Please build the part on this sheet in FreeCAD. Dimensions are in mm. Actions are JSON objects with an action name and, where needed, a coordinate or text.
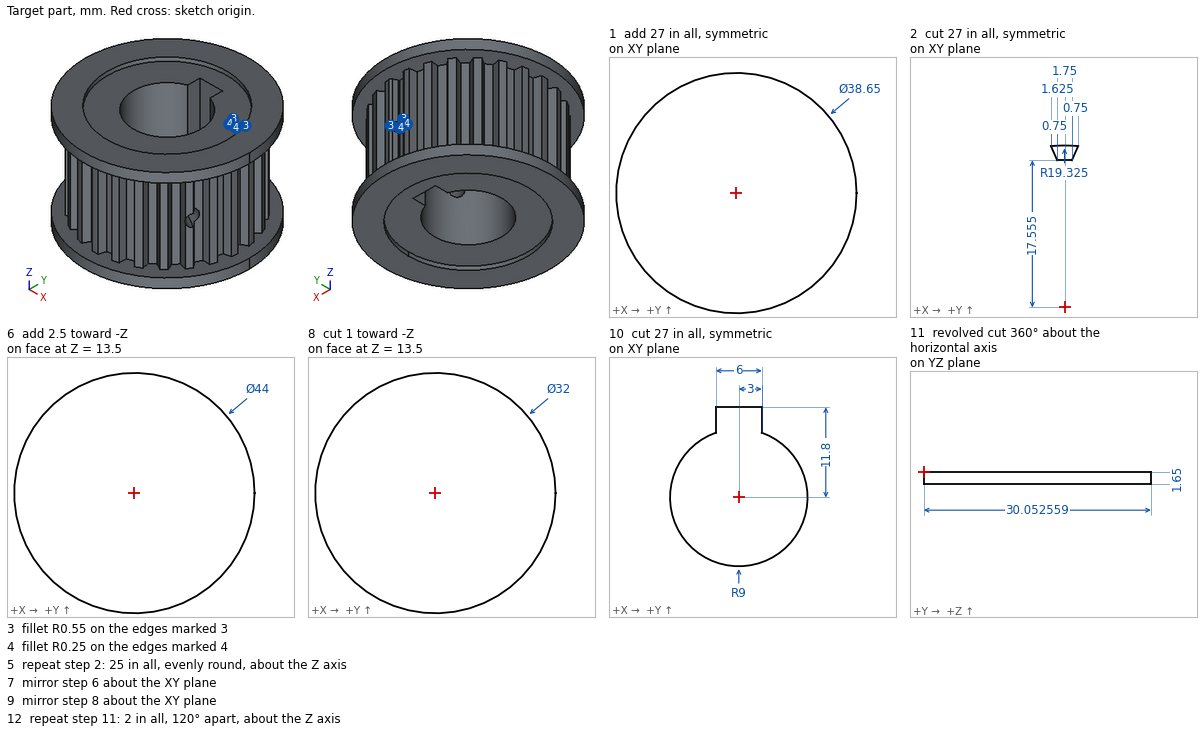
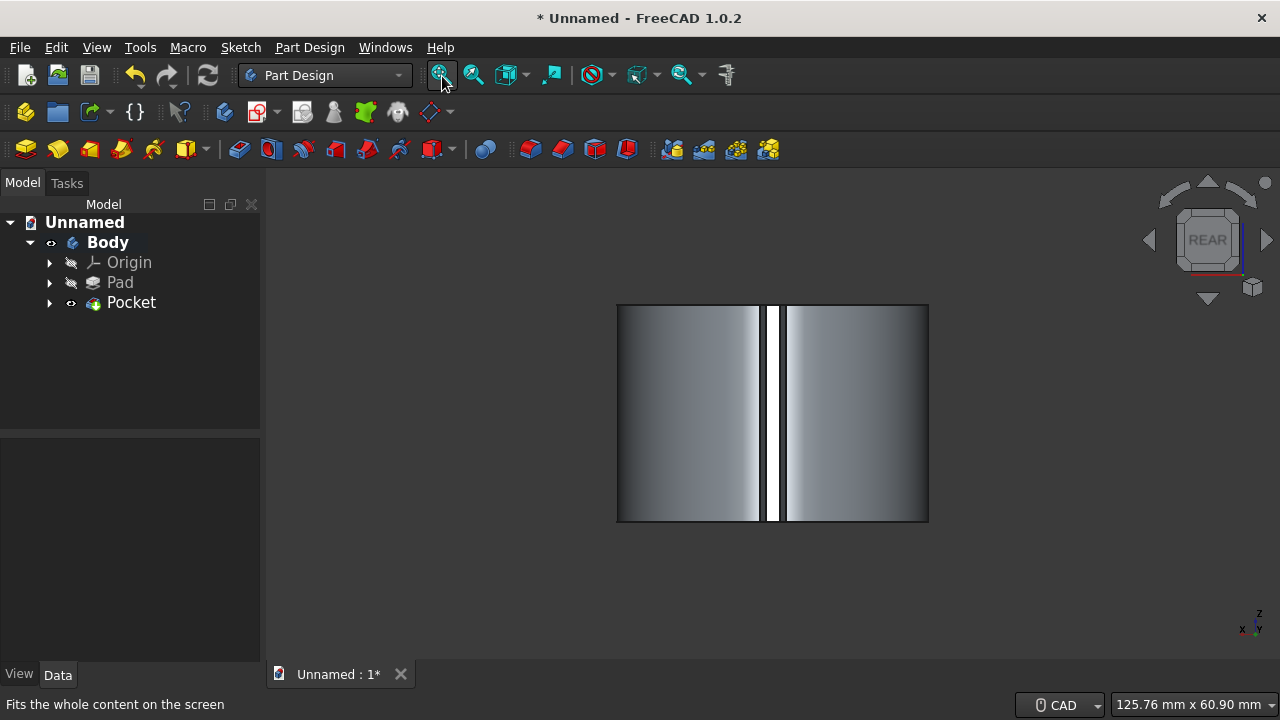
{"action": "left_click", "coordinate": [442, 76]}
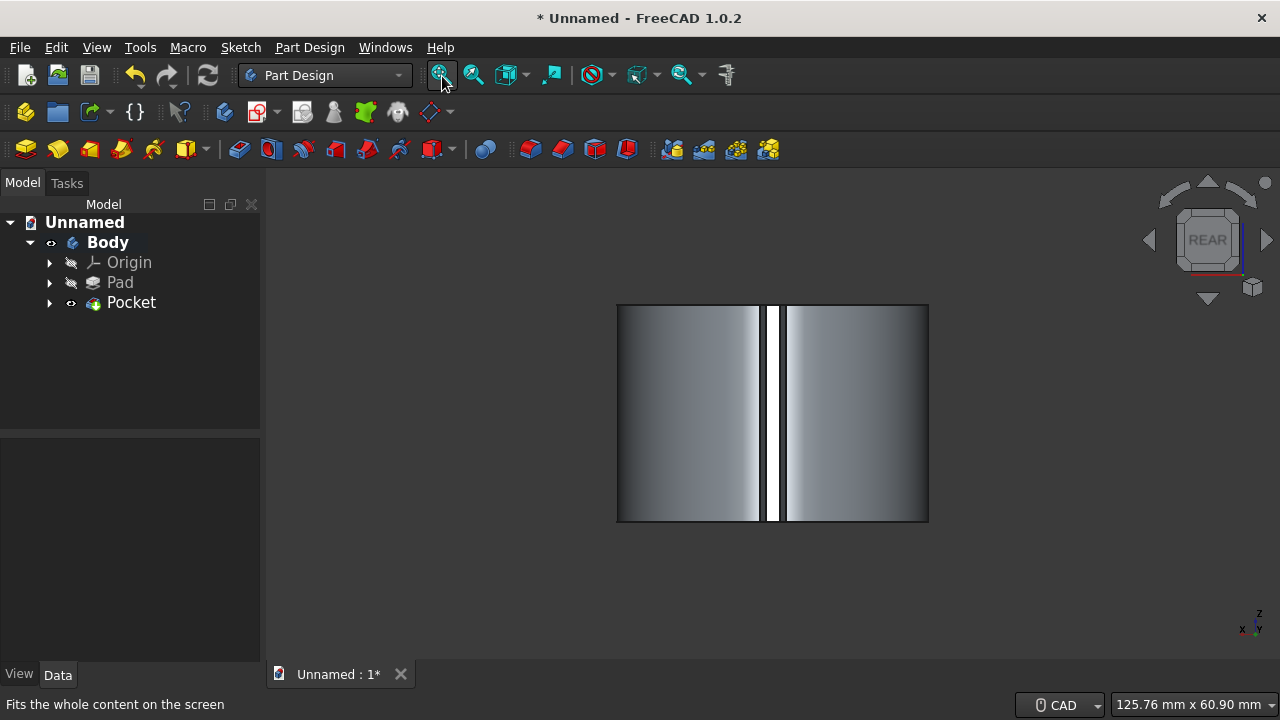
{"action": "left_click", "coordinate": [786, 413]}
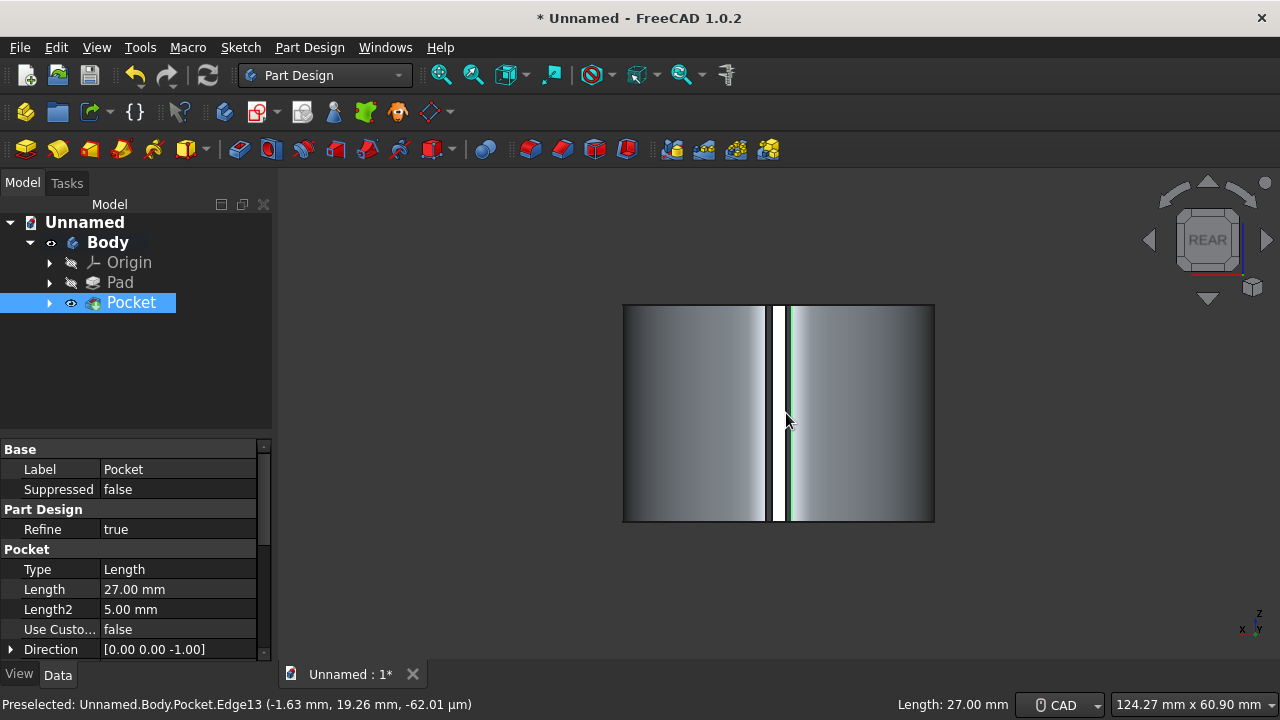
{"action": "left_click", "coordinate": [766, 413], "text": "ctrl"}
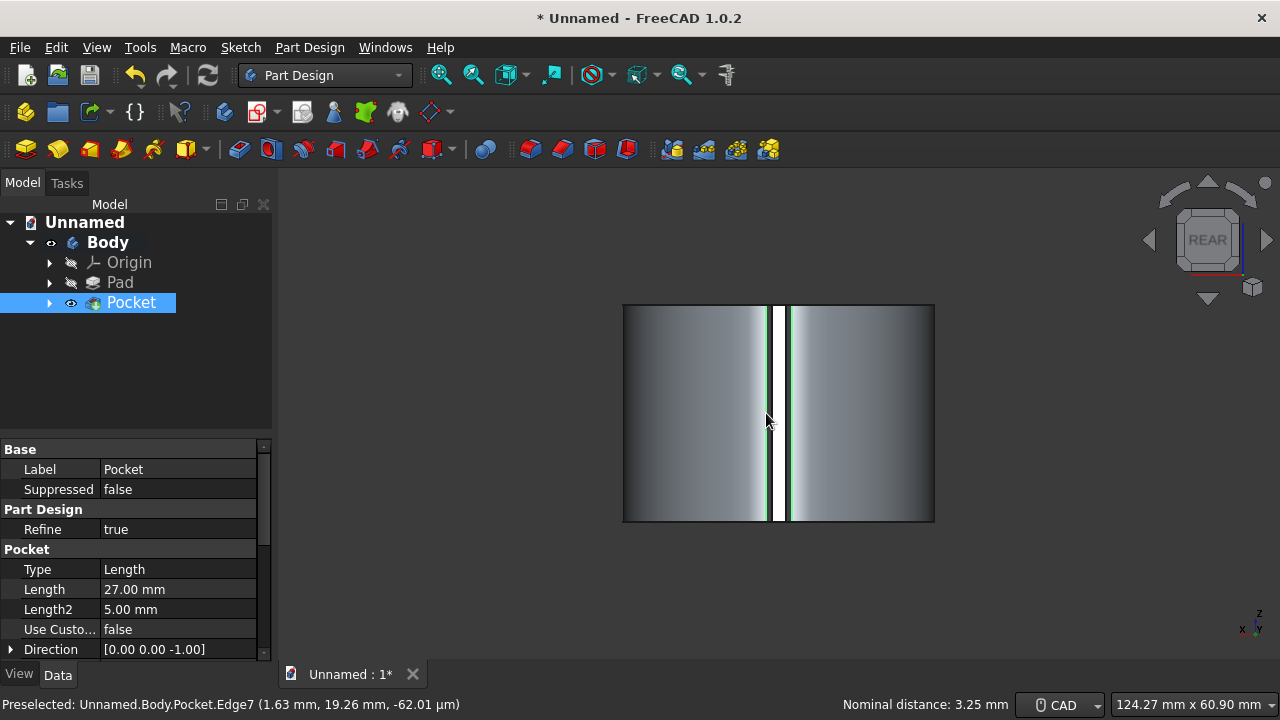
{"action": "left_click", "coordinate": [532, 150]}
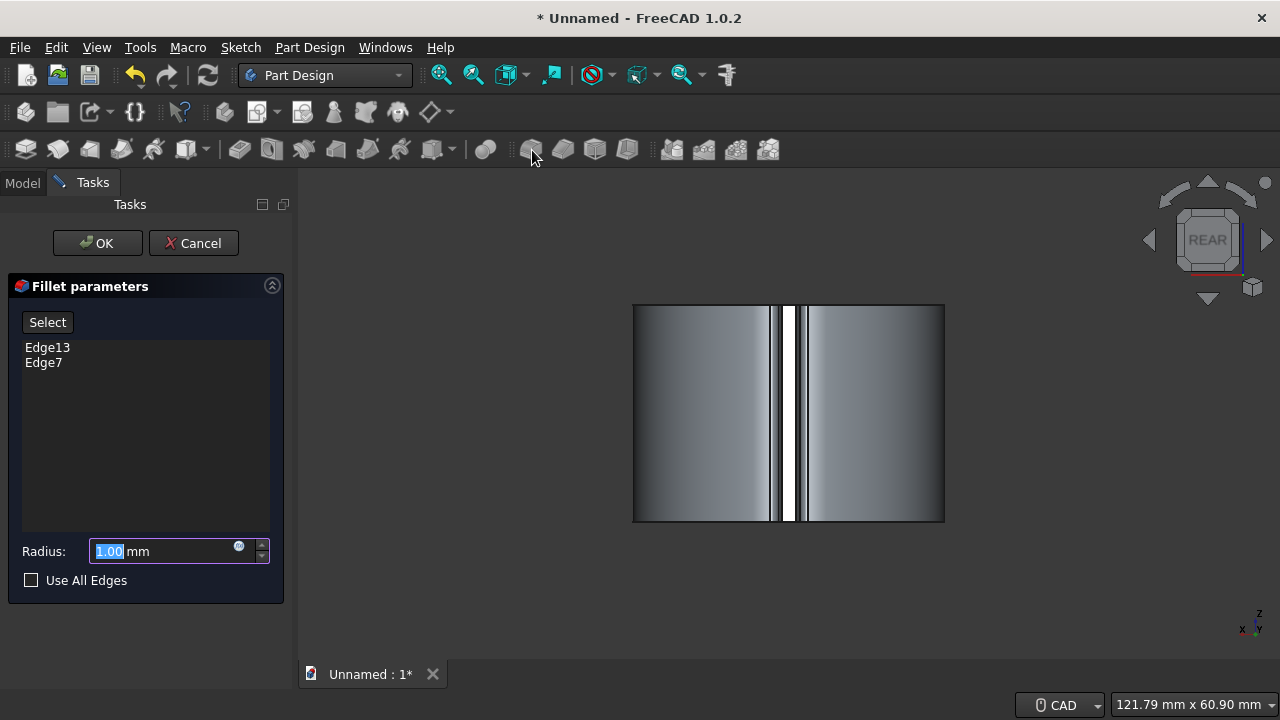
{"action": "type", "text": "0.55"}
{"action": "key", "text": "Tab"}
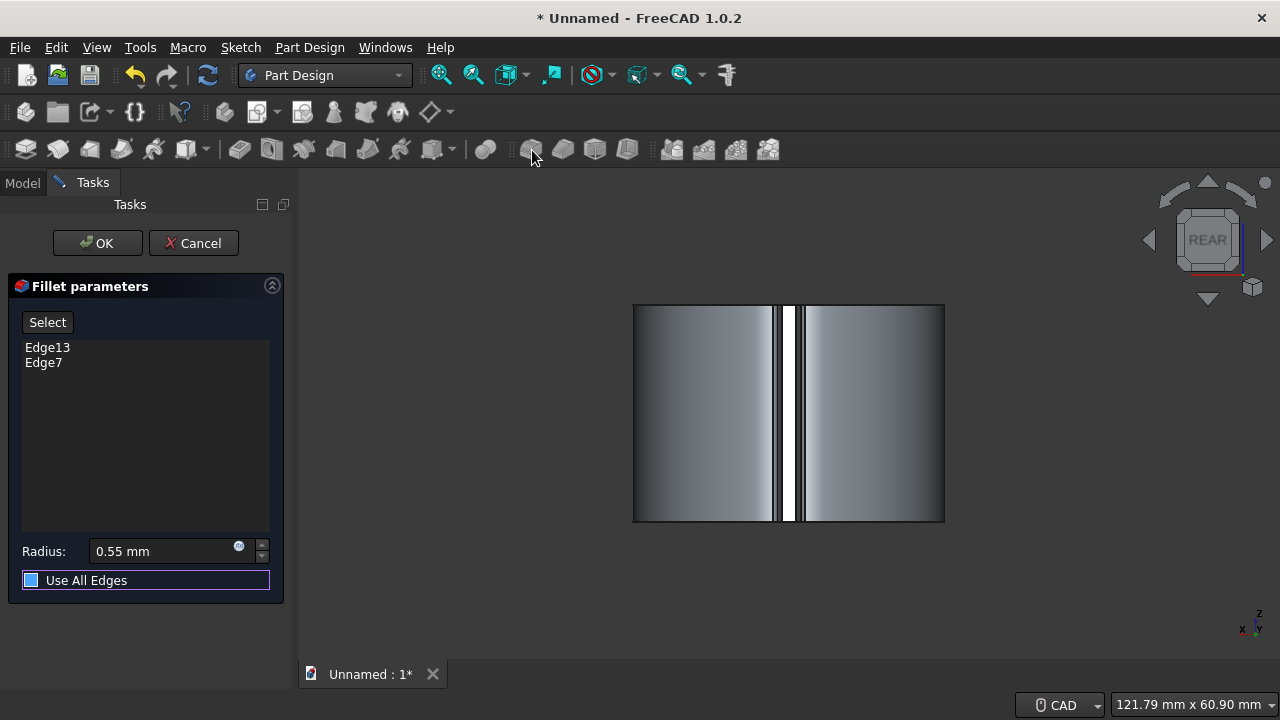
{"action": "left_click", "coordinate": [98, 243]}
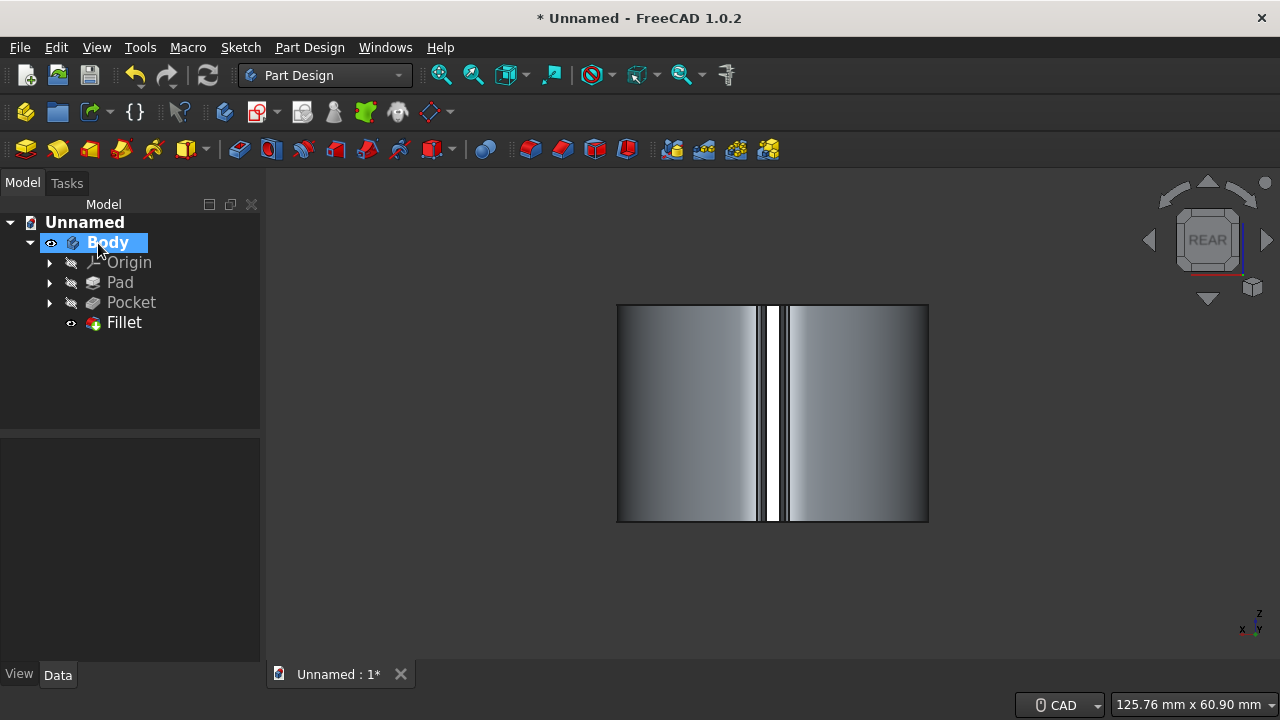
{"action": "left_click", "coordinate": [442, 76]}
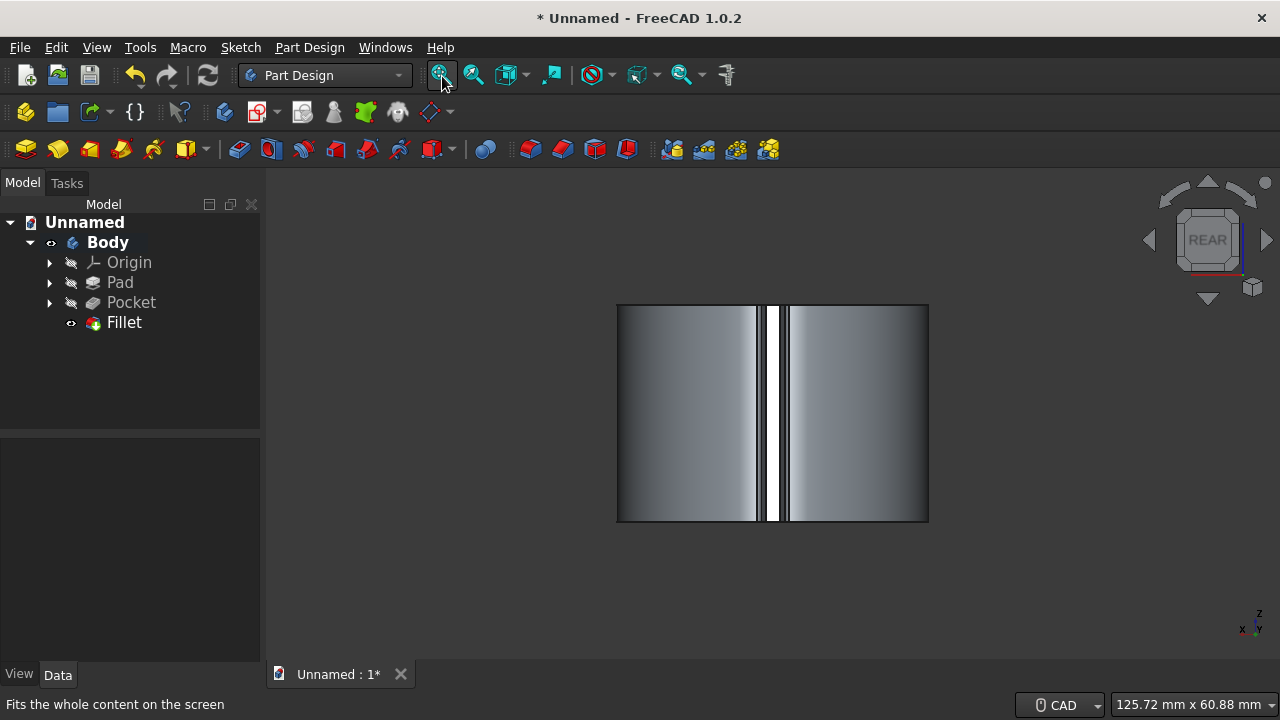
{"action": "key", "text": "0"}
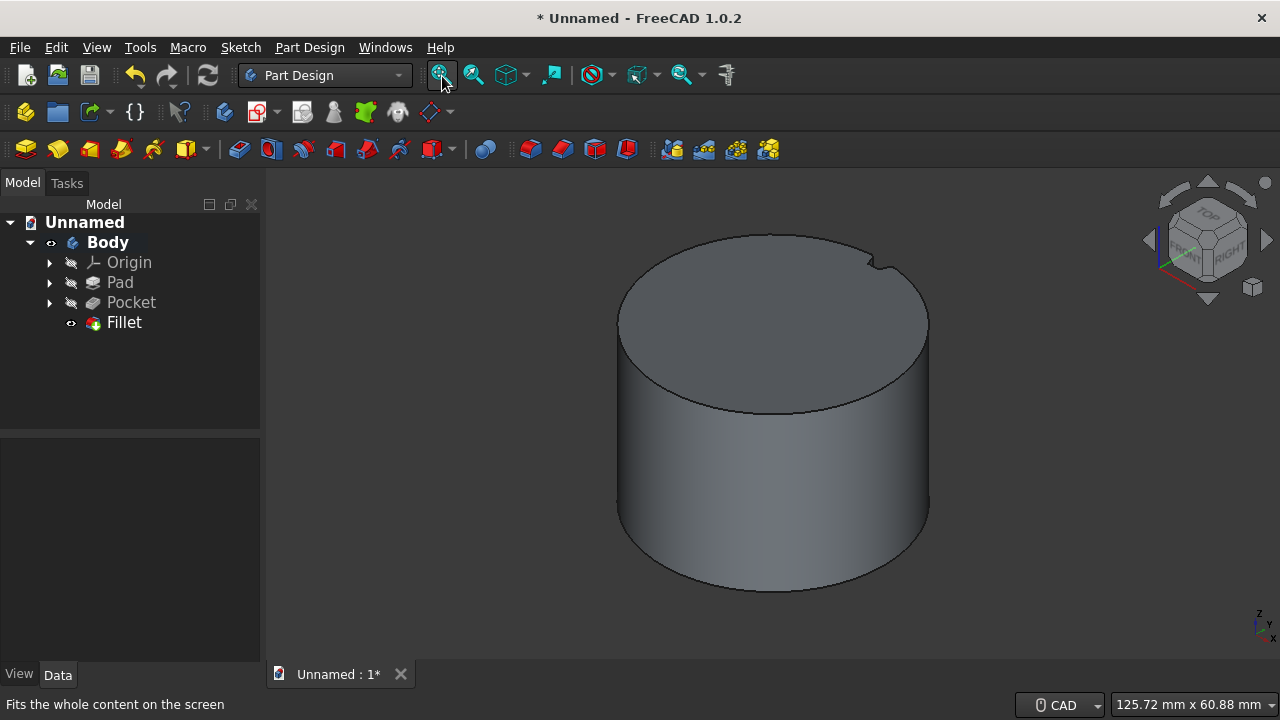
{"action": "key", "text": "2"}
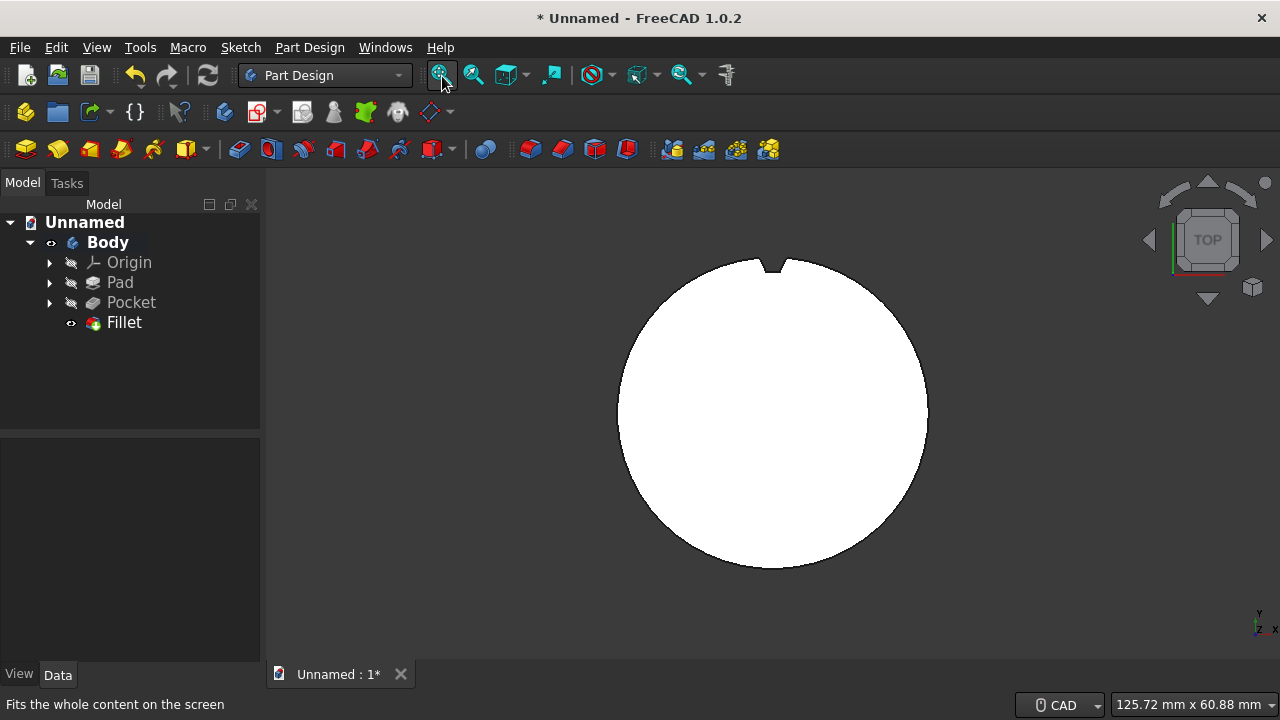
{"action": "key", "text": "1"}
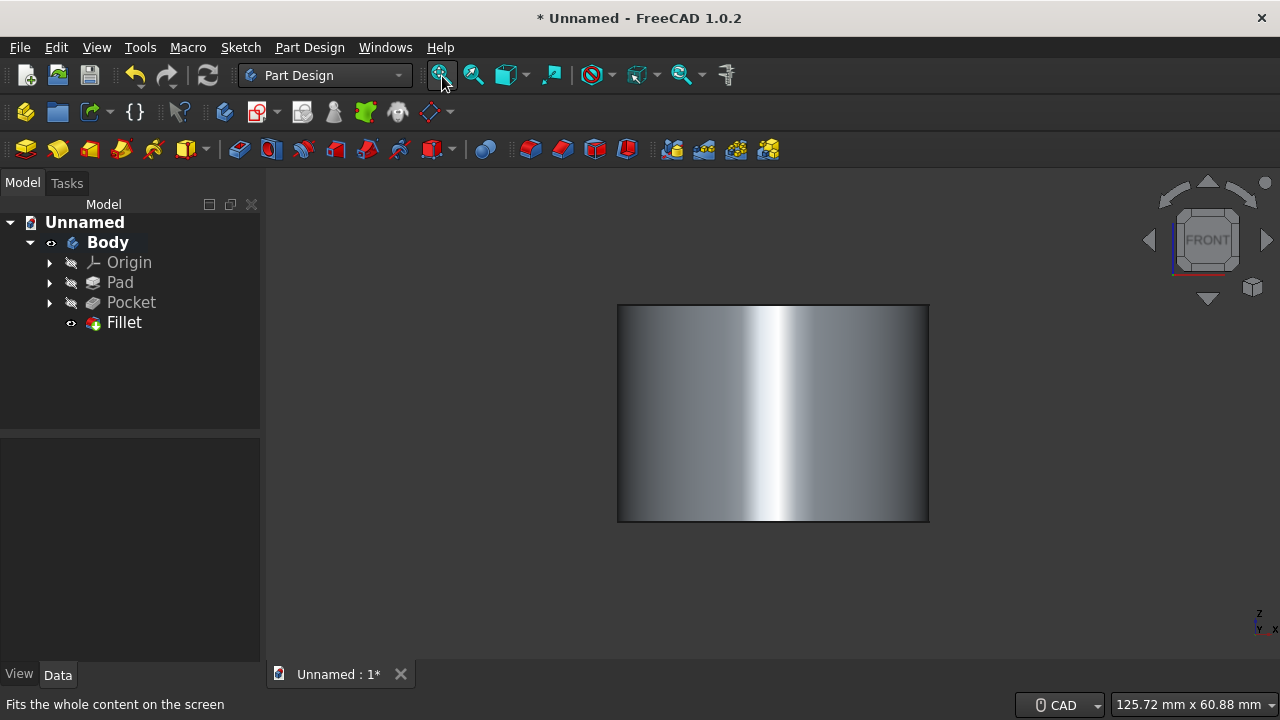
{"action": "left_click", "coordinate": [442, 76]}